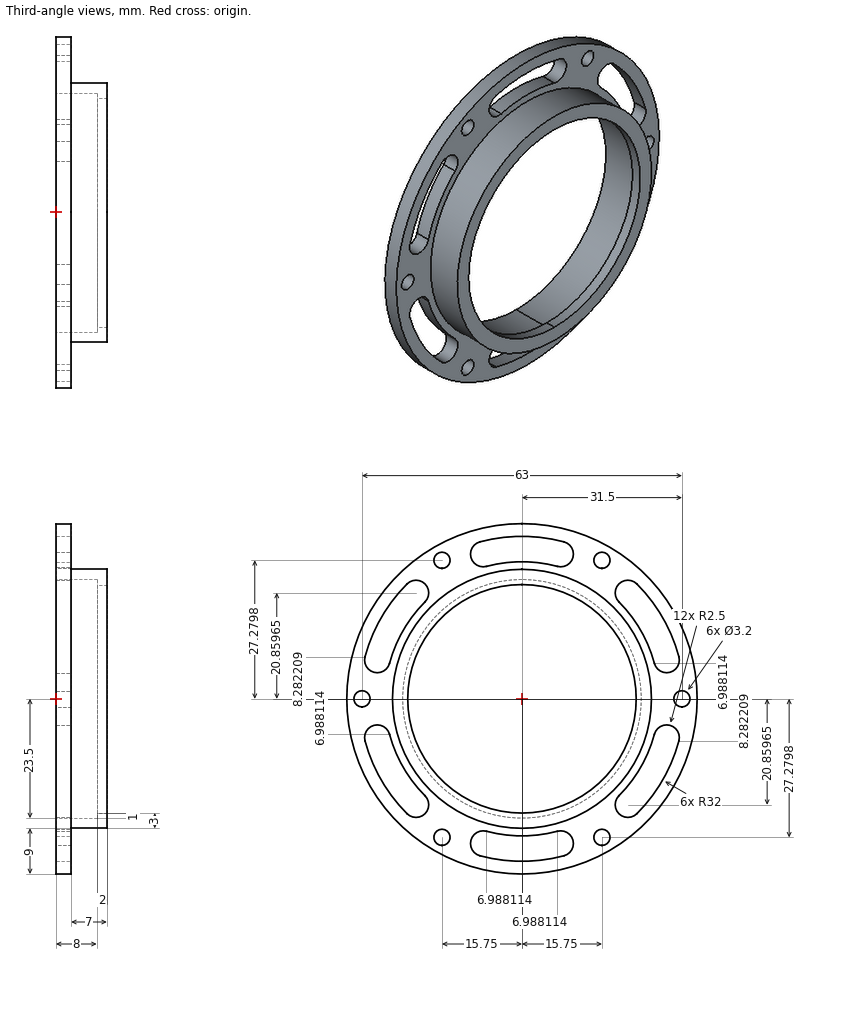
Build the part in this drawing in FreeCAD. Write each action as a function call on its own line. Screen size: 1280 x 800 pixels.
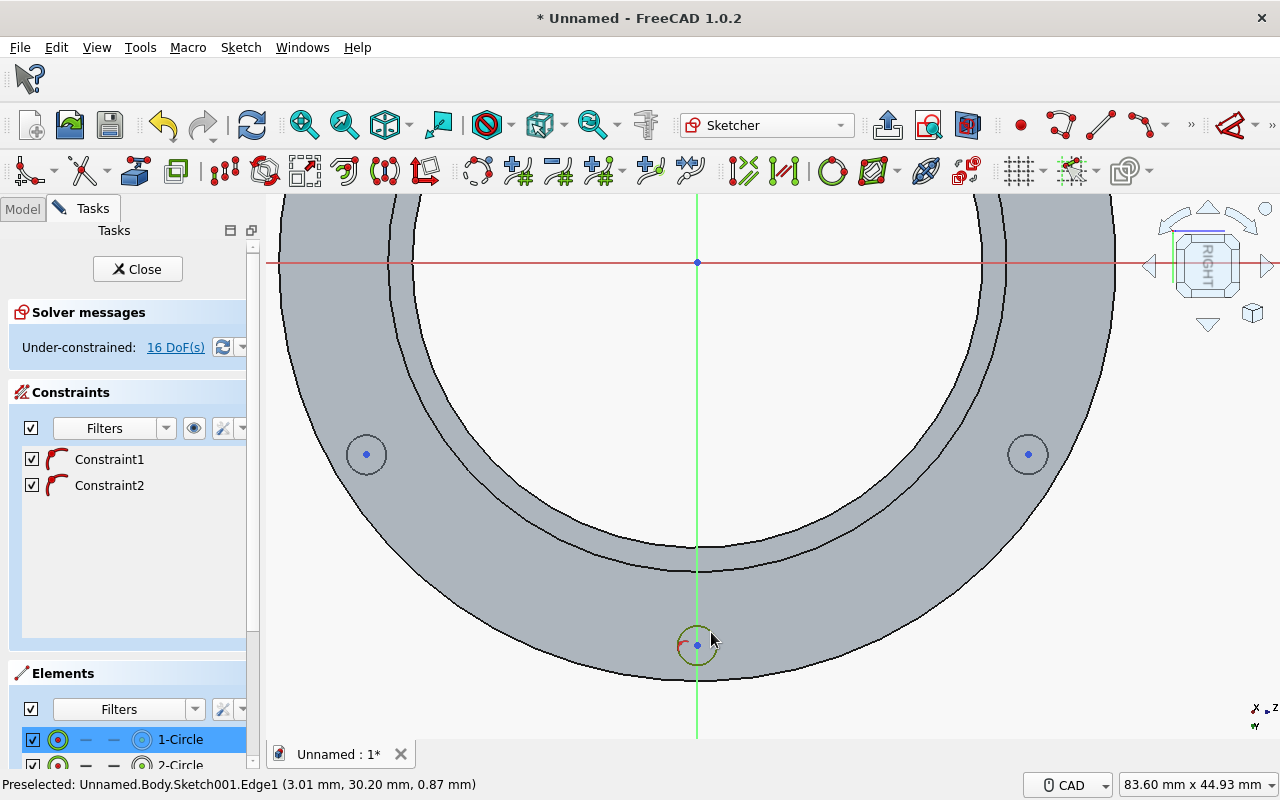
click(380, 441)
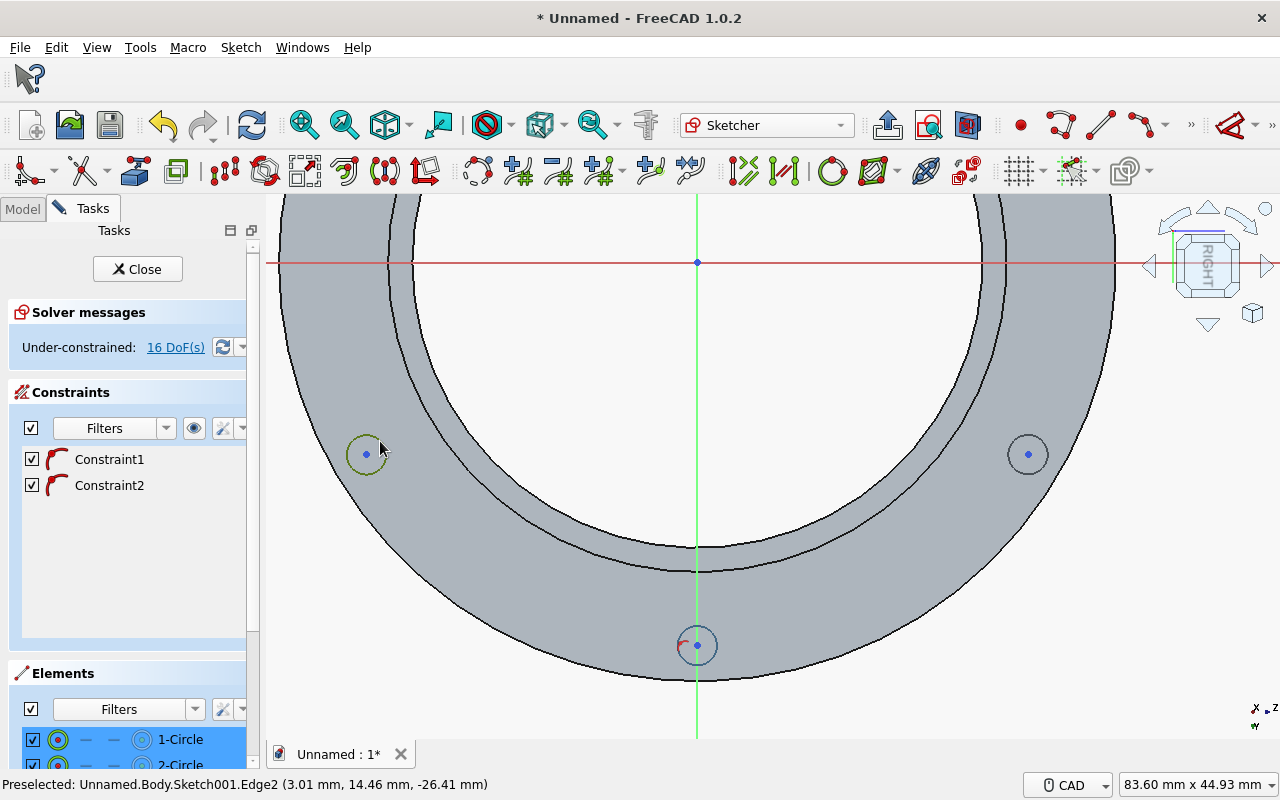
scroll(710, 633, down, 4)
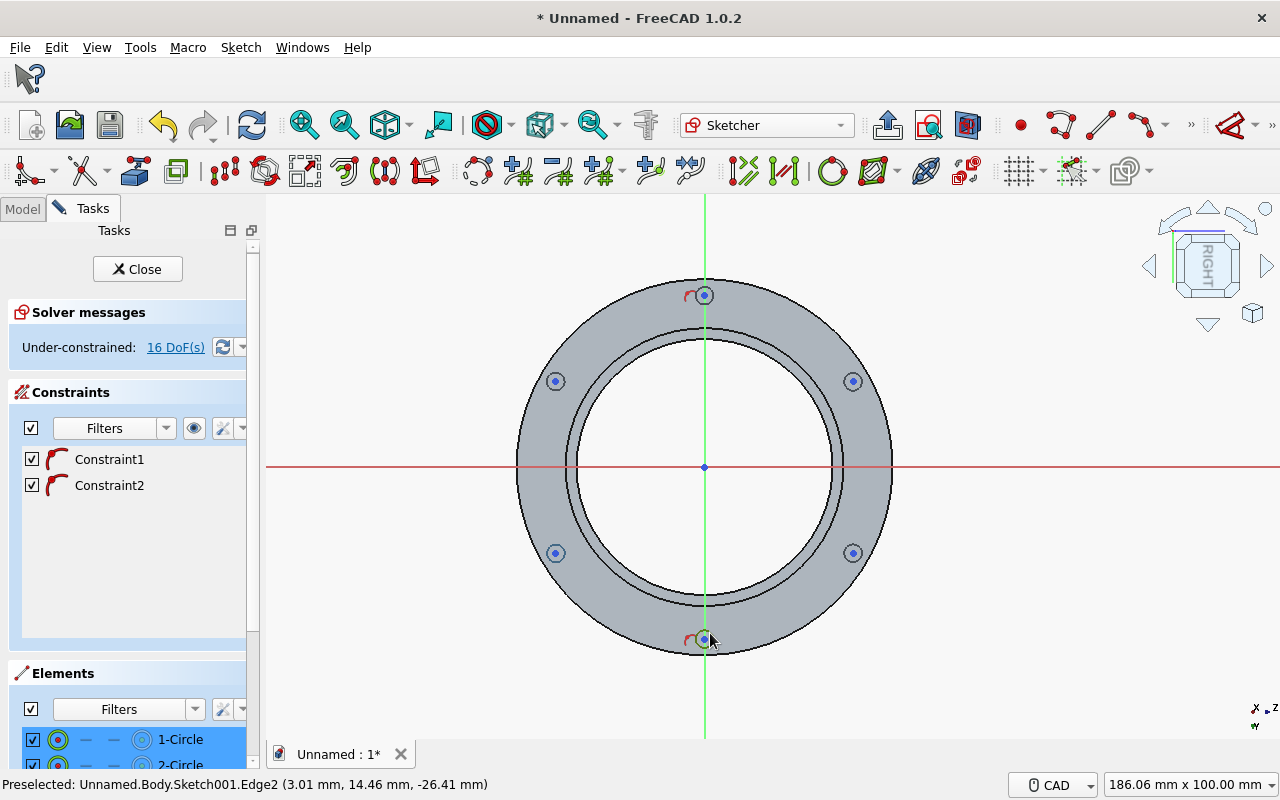
scroll(562, 375, up, 3)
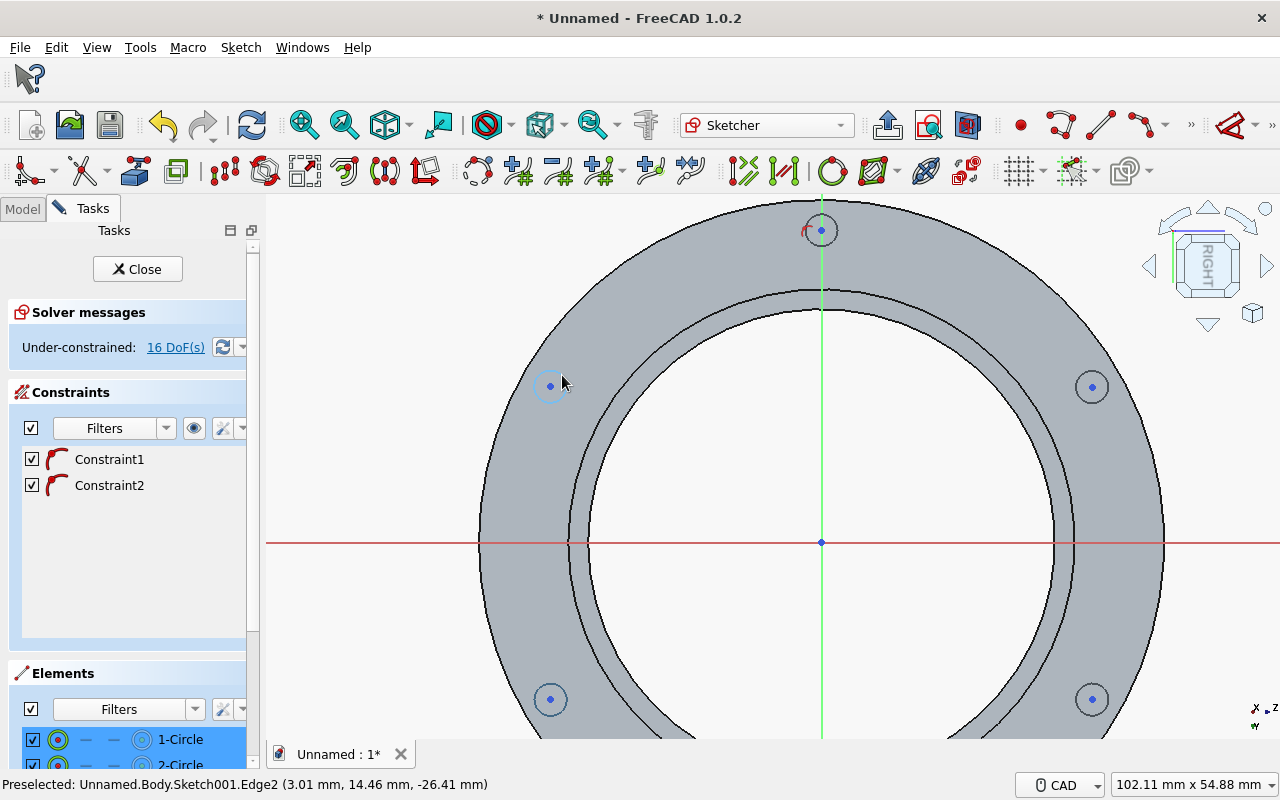
click(562, 375)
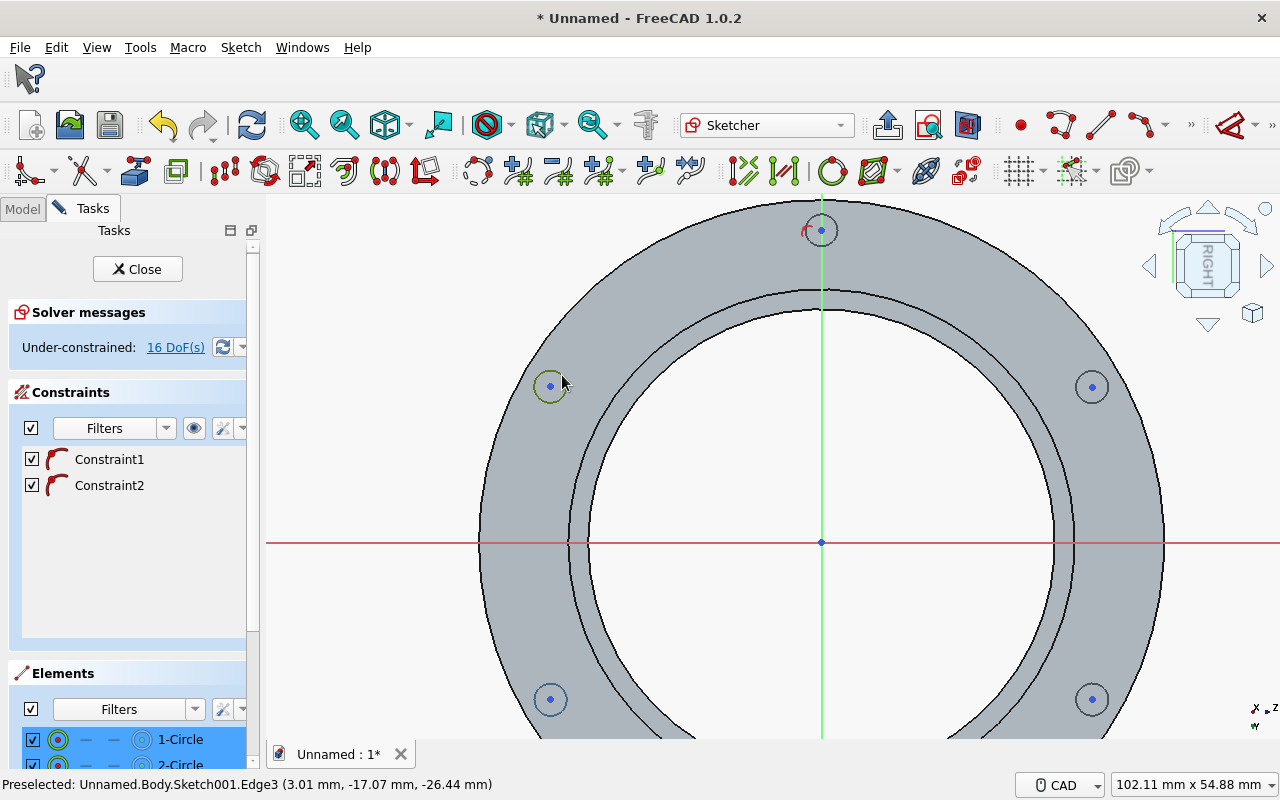
scroll(810, 242, up, 2)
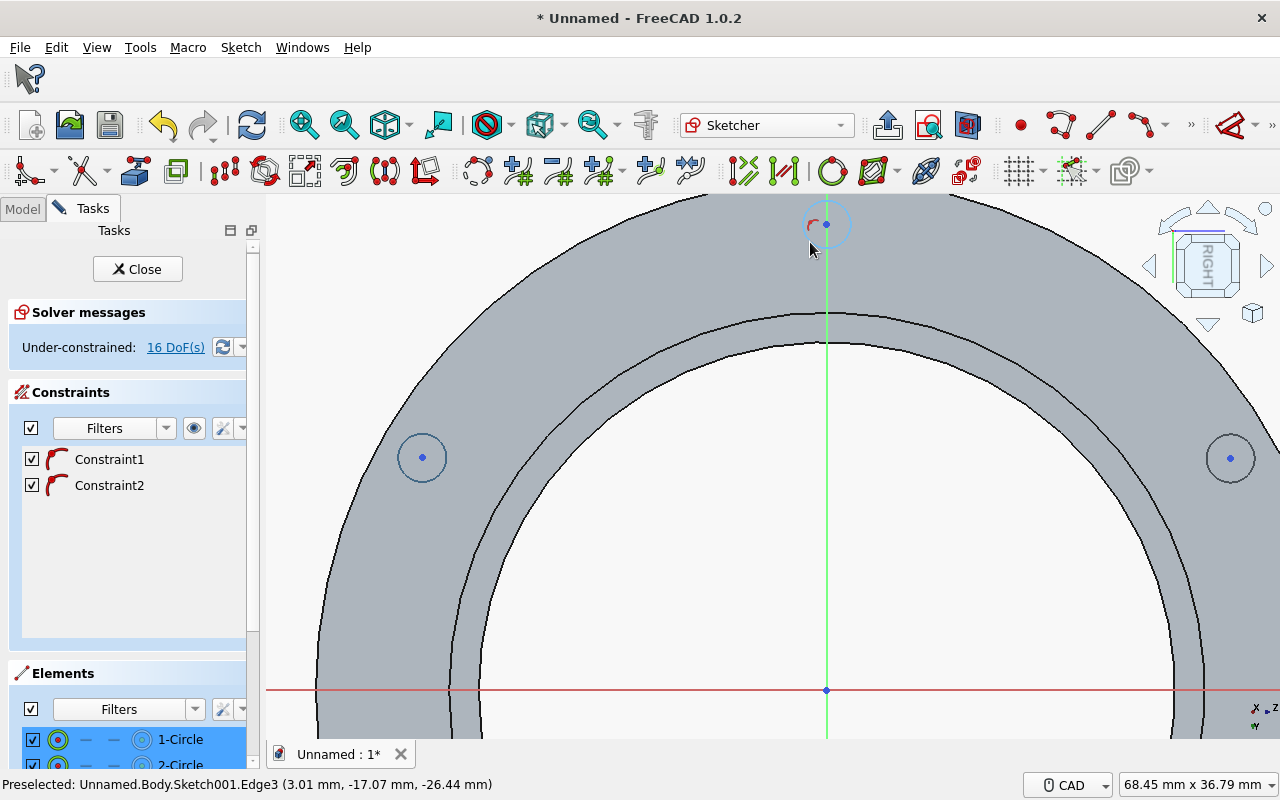
click(810, 241)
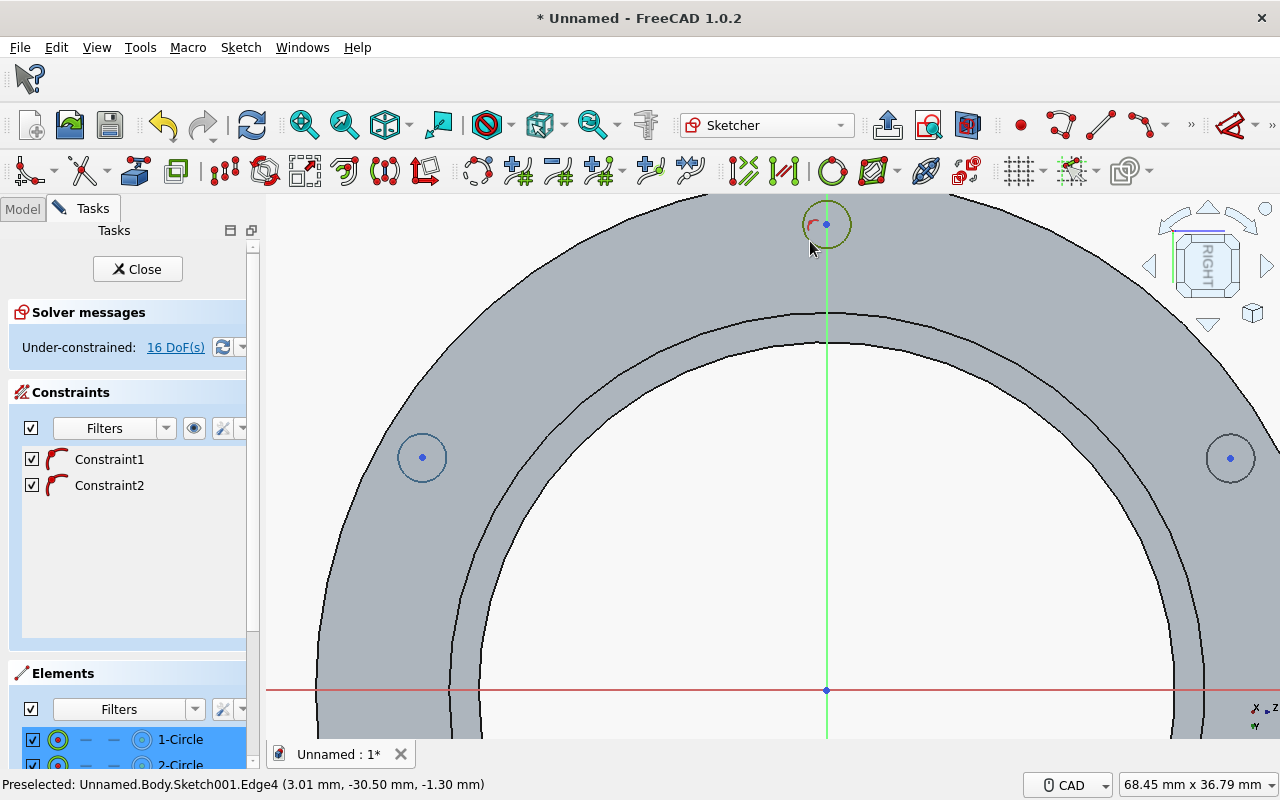
scroll(633, 336, down, 5)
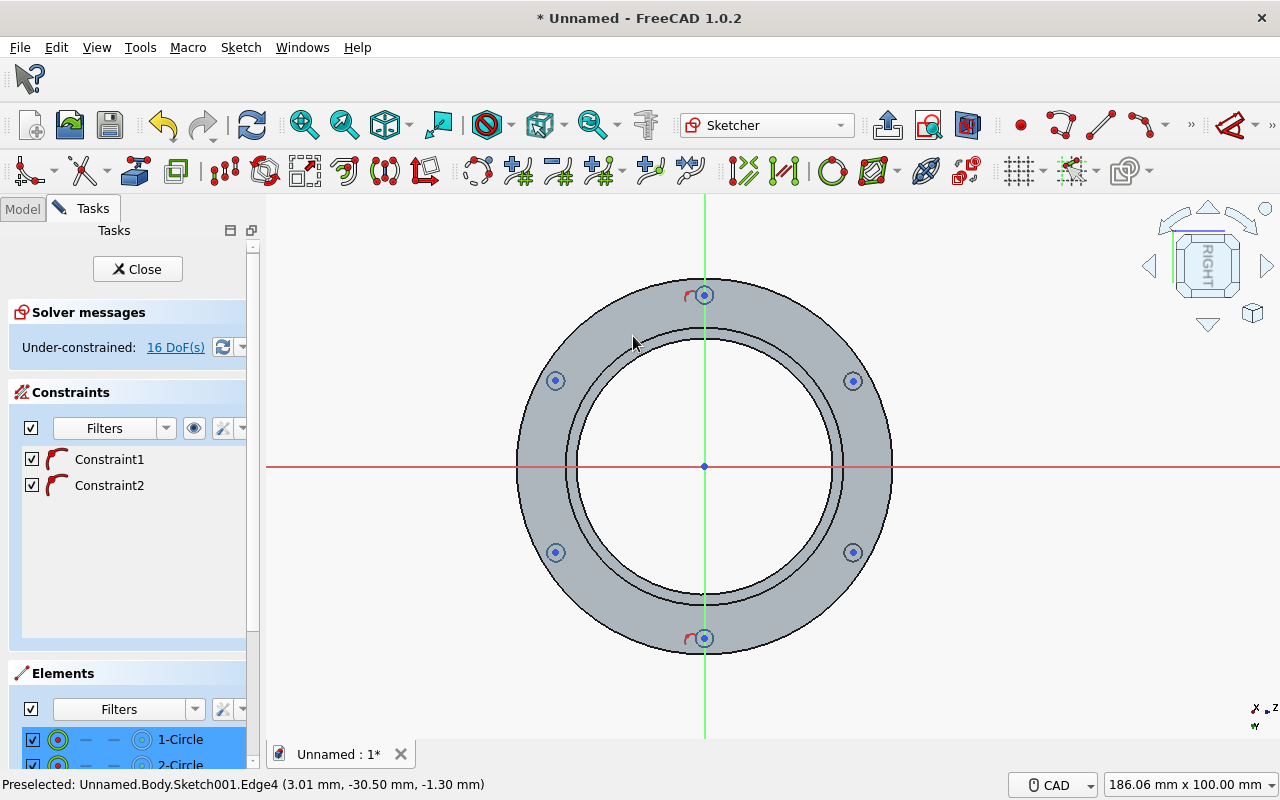
scroll(859, 375, up, 3)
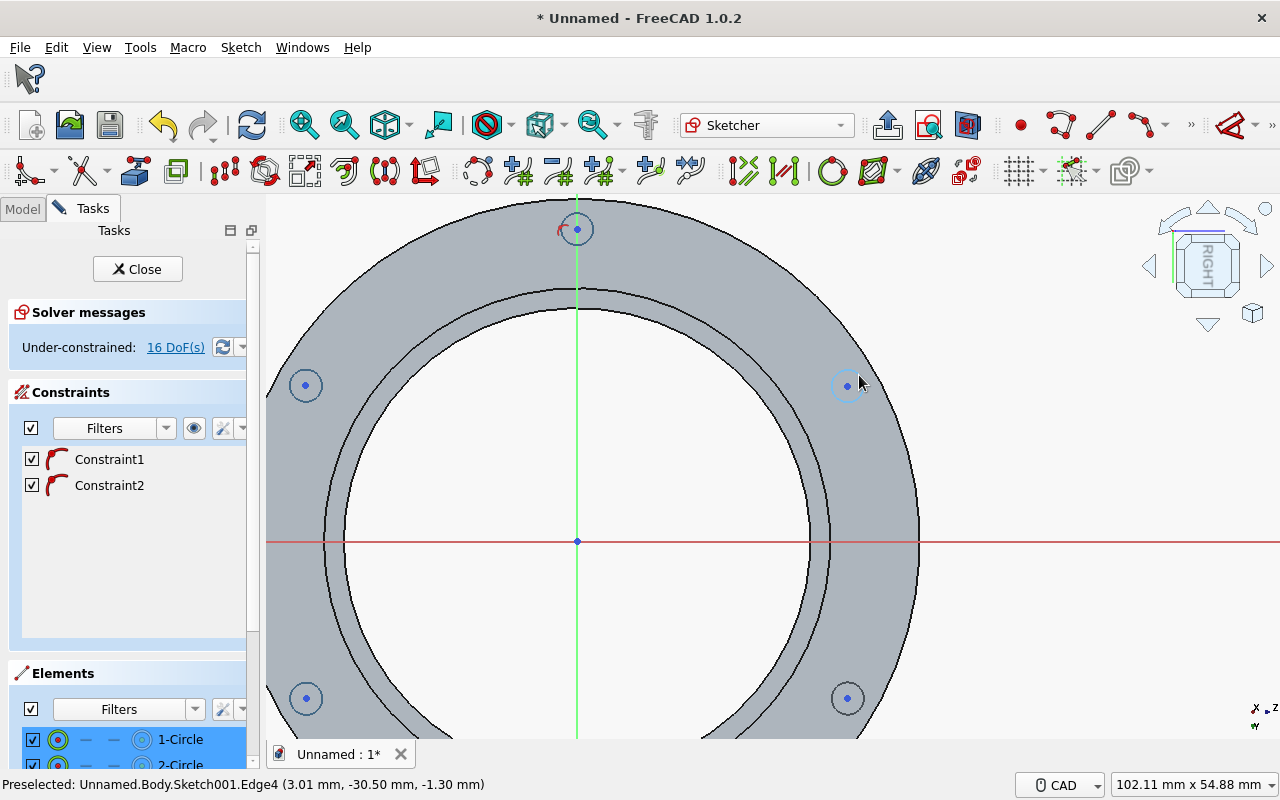
click(859, 375)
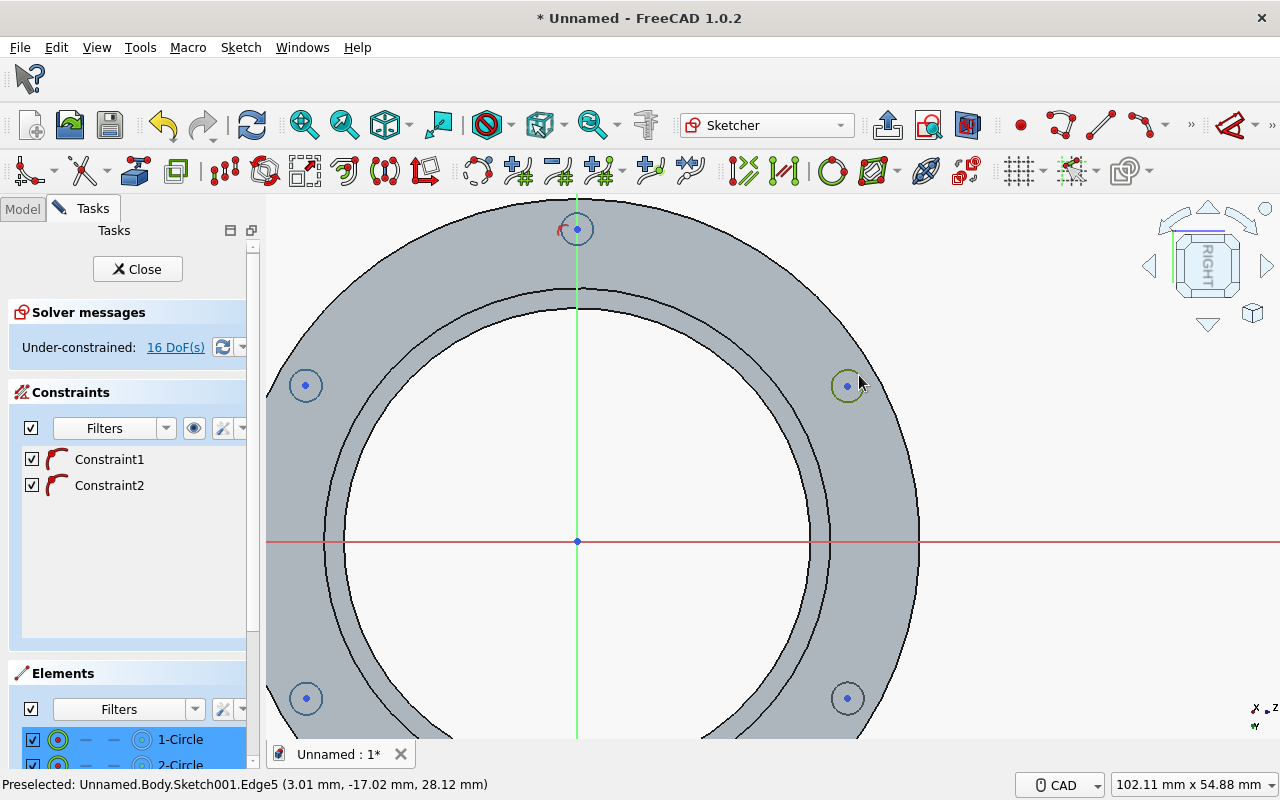
click(859, 687)